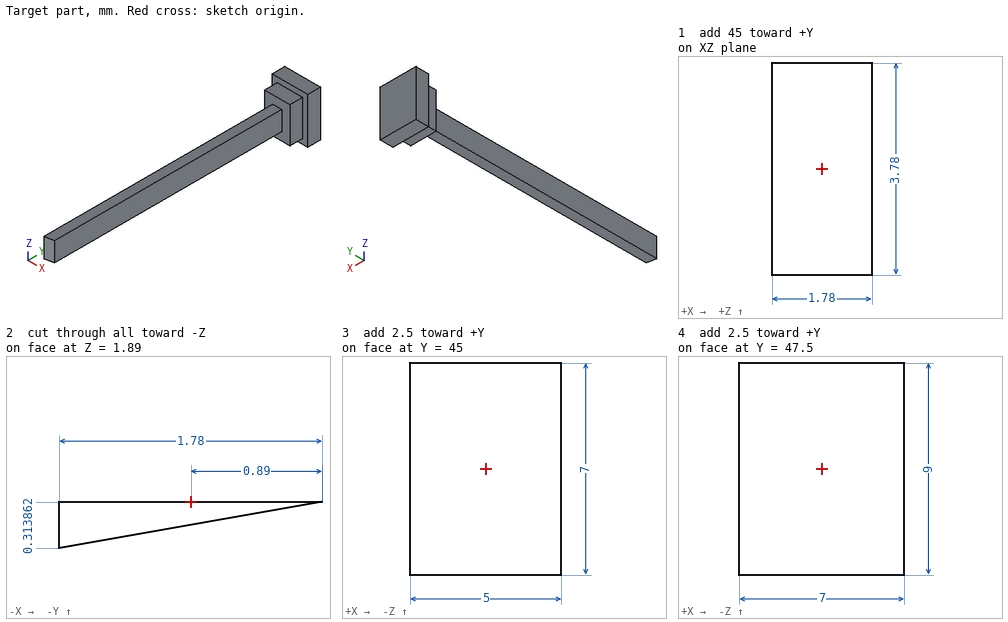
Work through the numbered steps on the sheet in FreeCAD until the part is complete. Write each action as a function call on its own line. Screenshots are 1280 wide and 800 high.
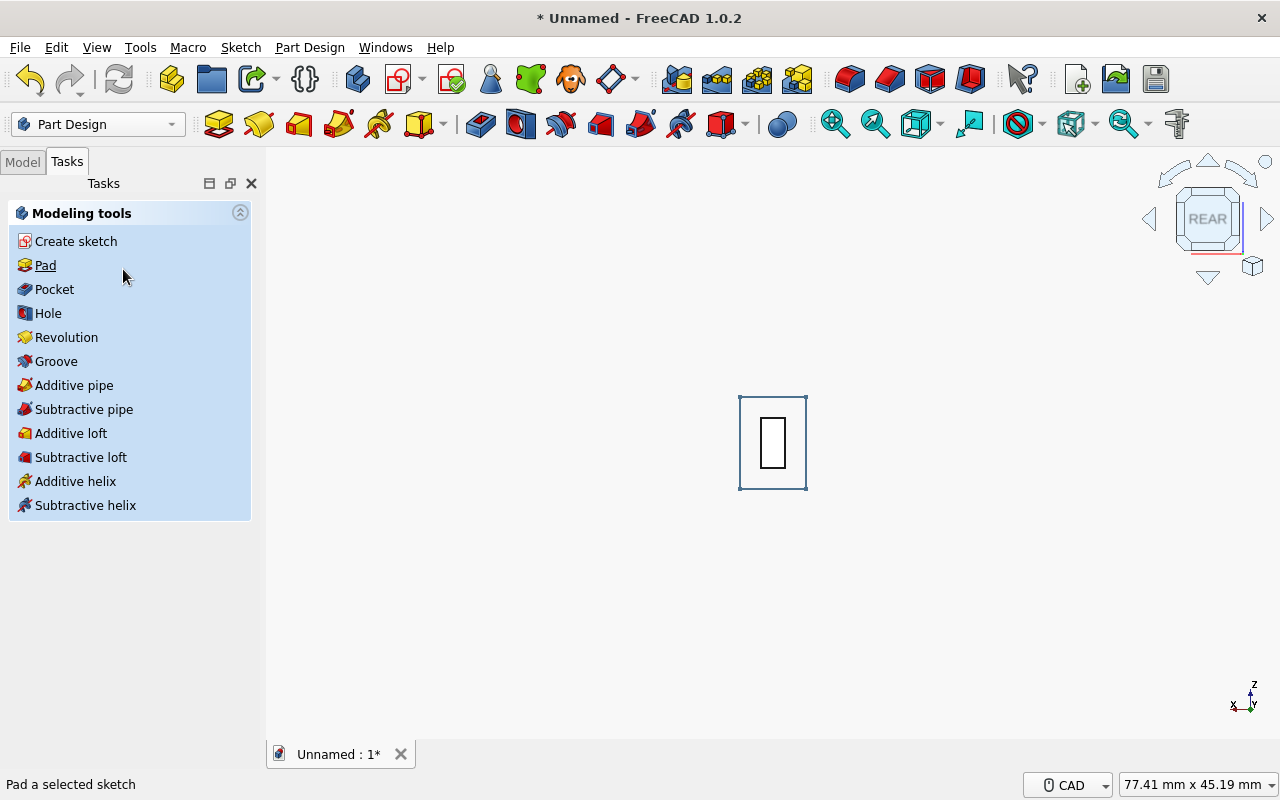
click(220, 124)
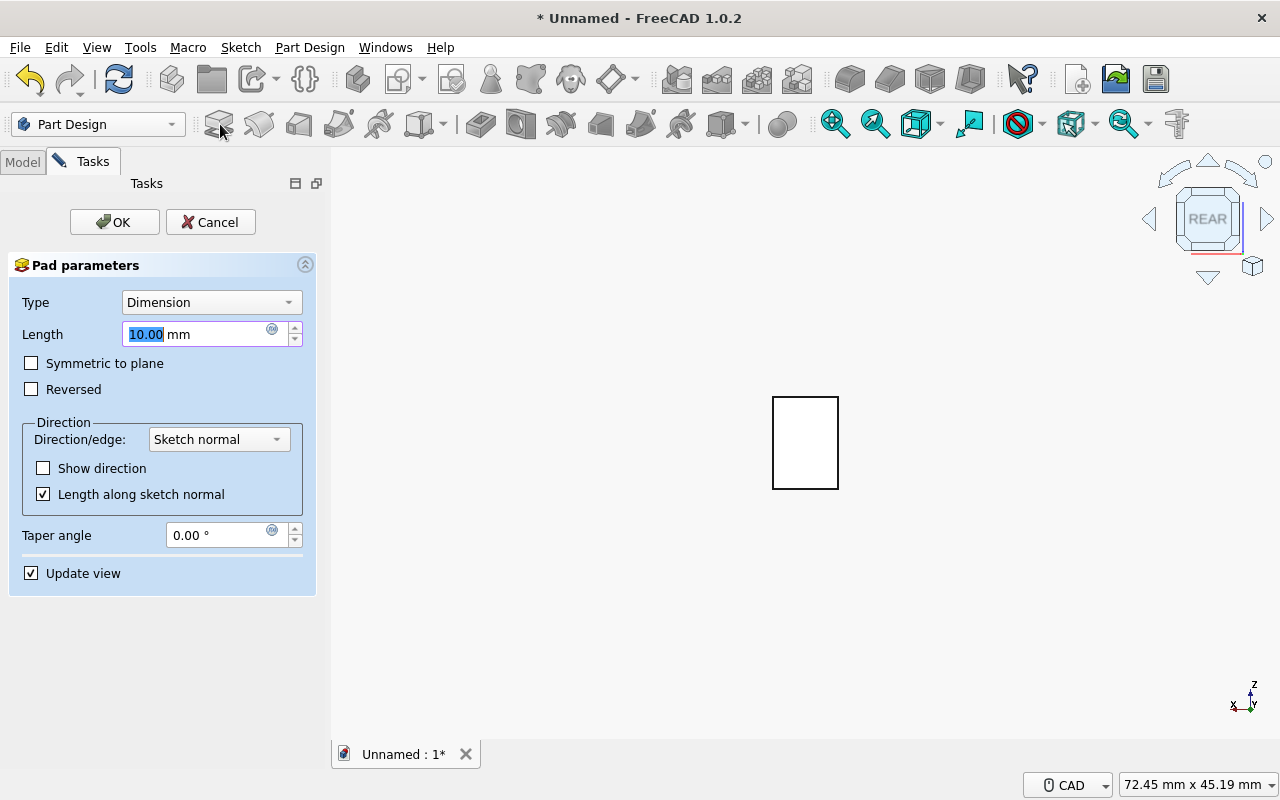
text(2.5)
key(Tab)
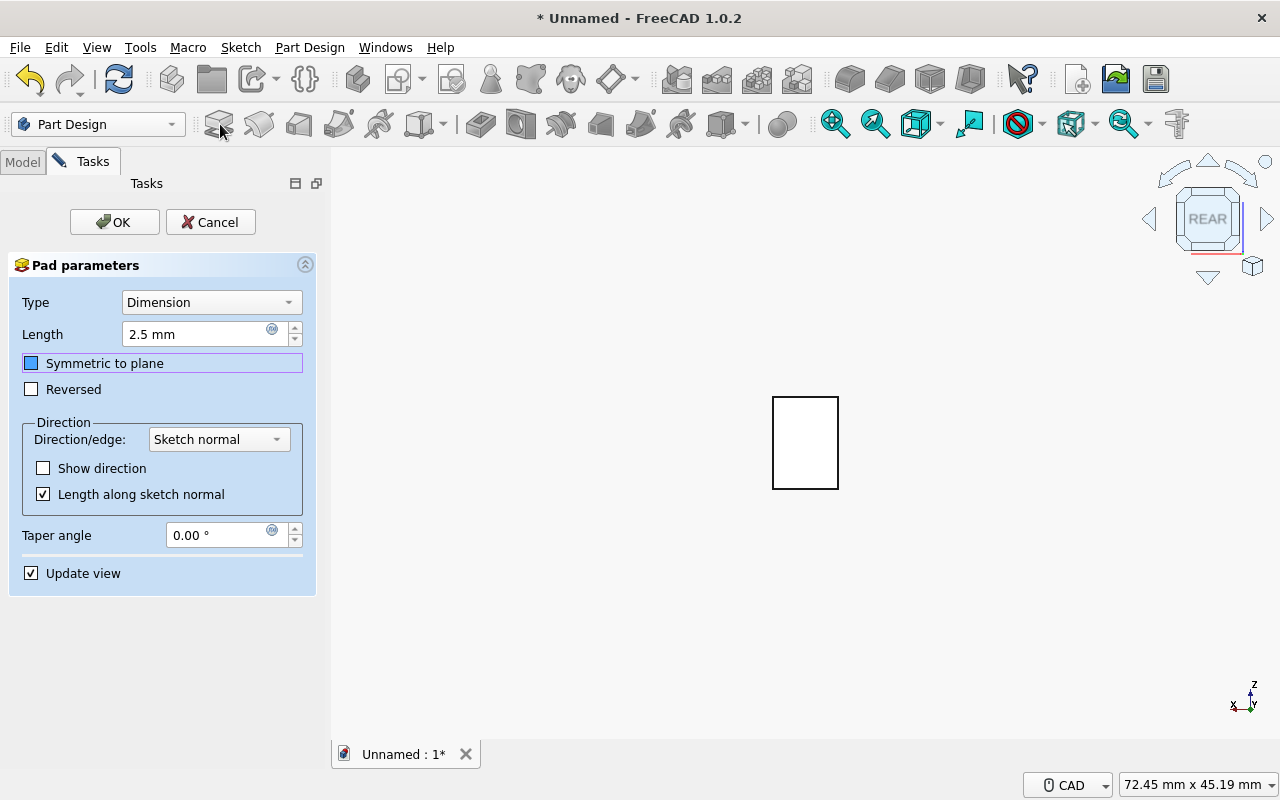
click(115, 222)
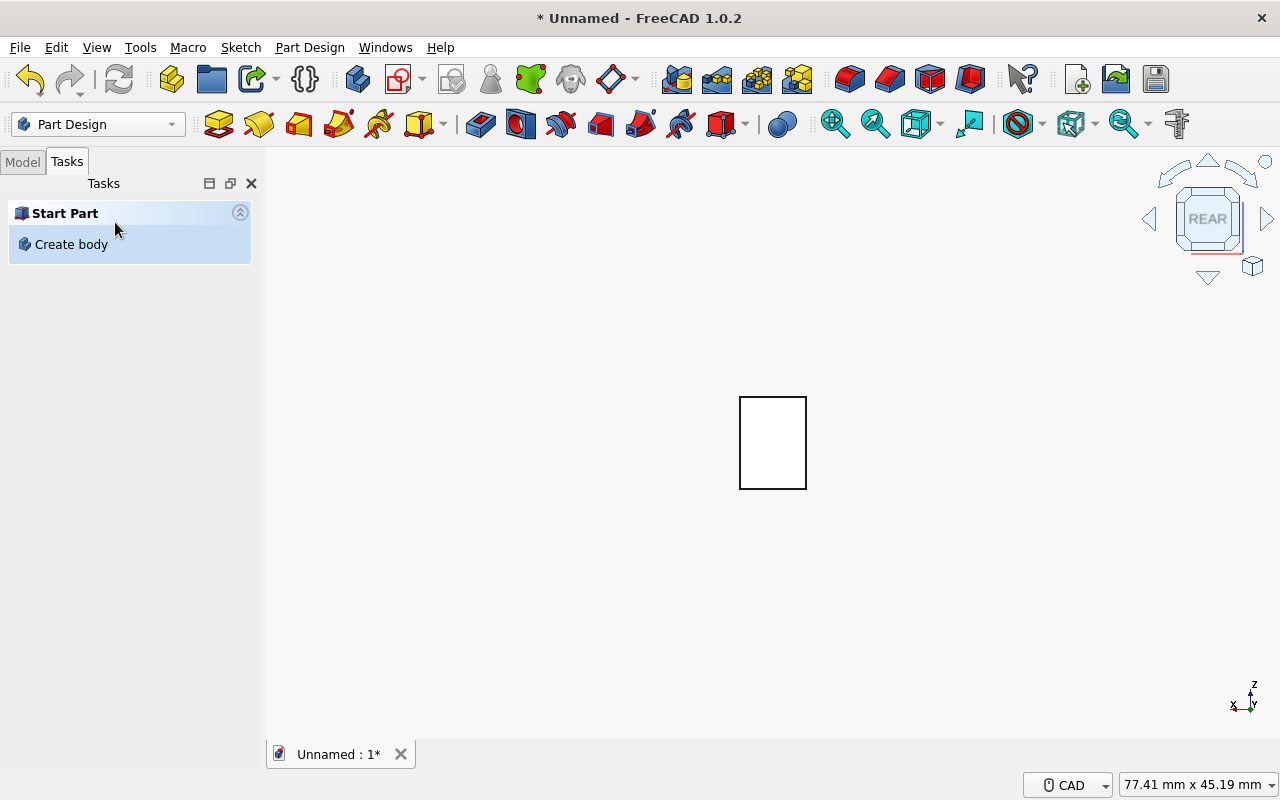
key(v)
key(f)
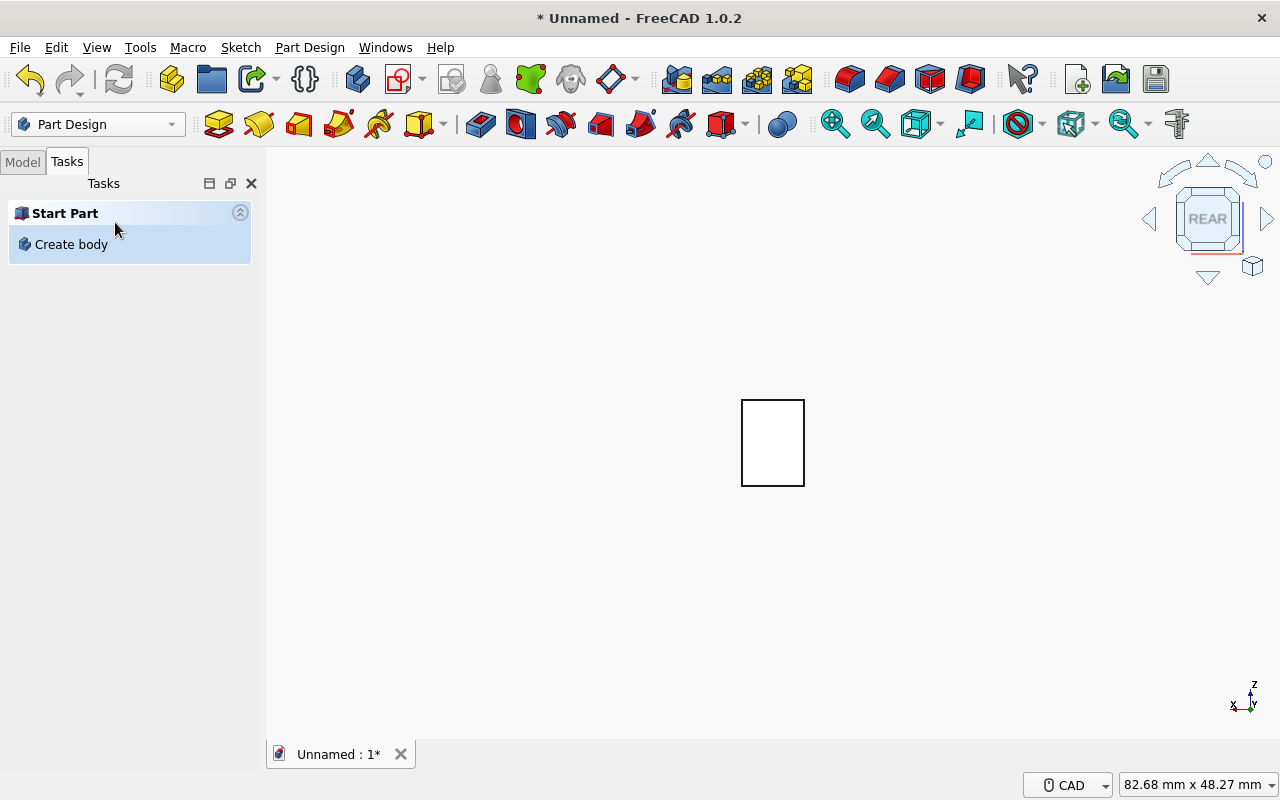
click(773, 430)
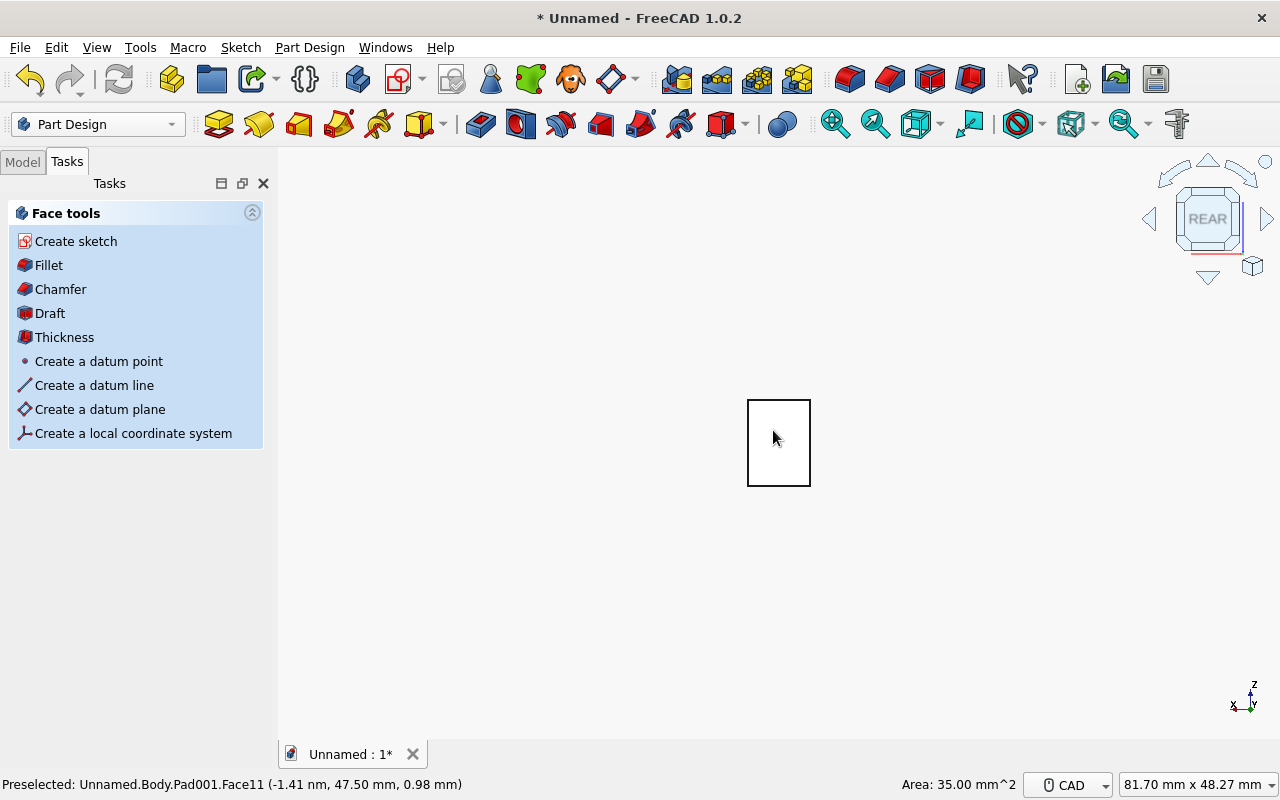
click(398, 80)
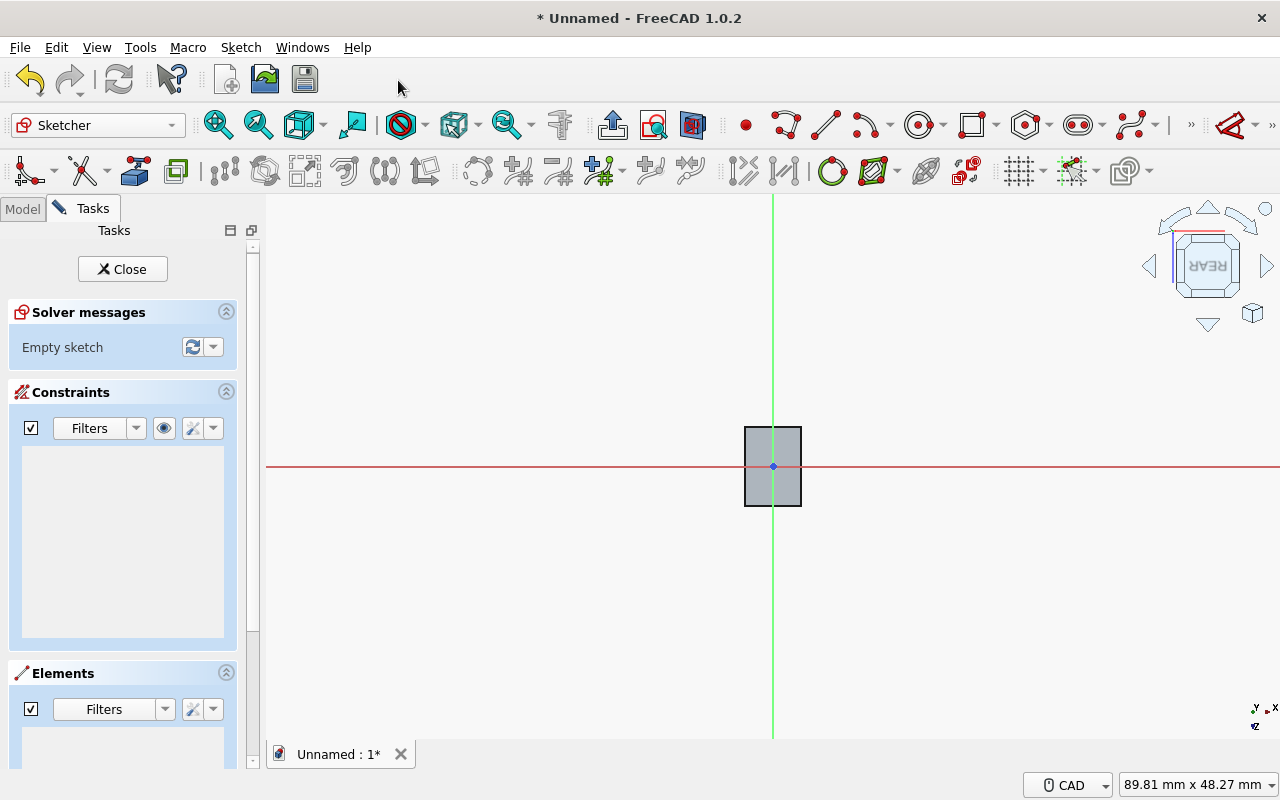
scroll(803, 466, up, 6)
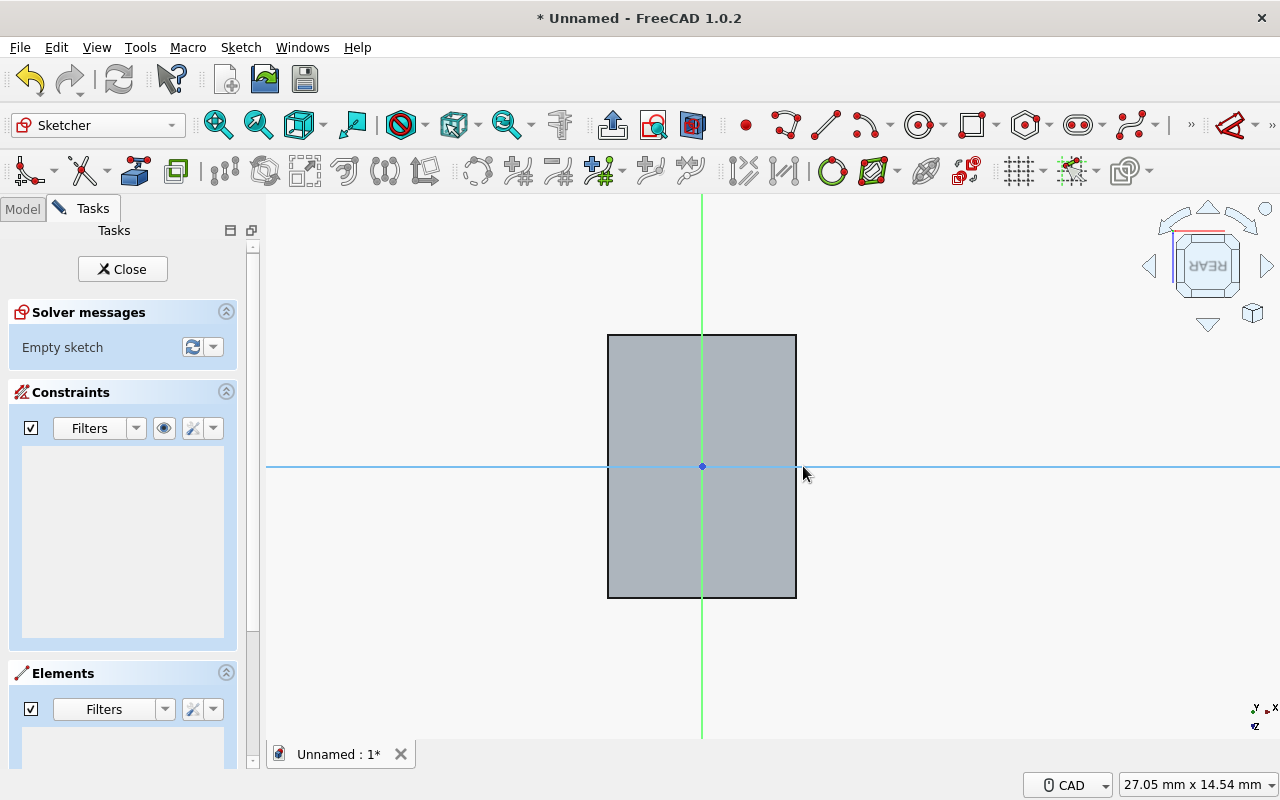
key(g)
key(v)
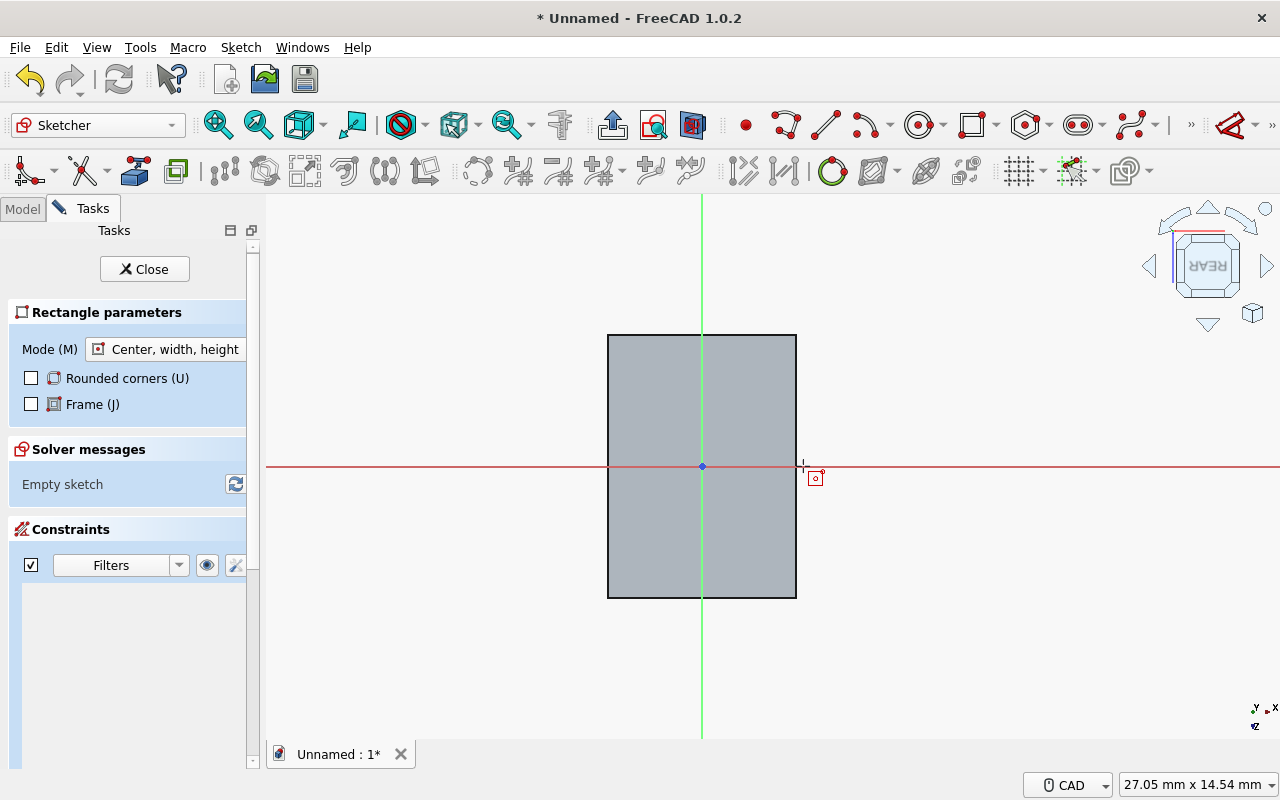
click(702, 466)
click(833, 298)
key(Escape)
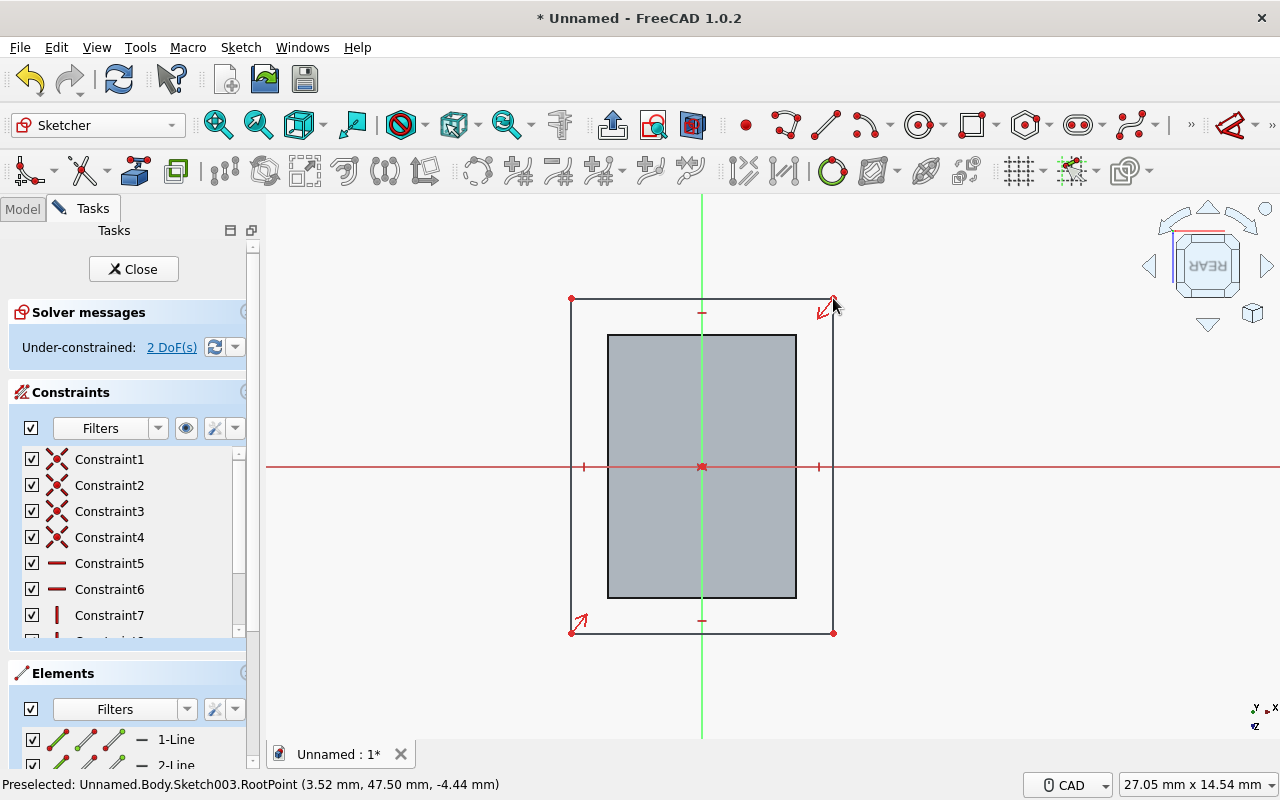
click(1230, 126)